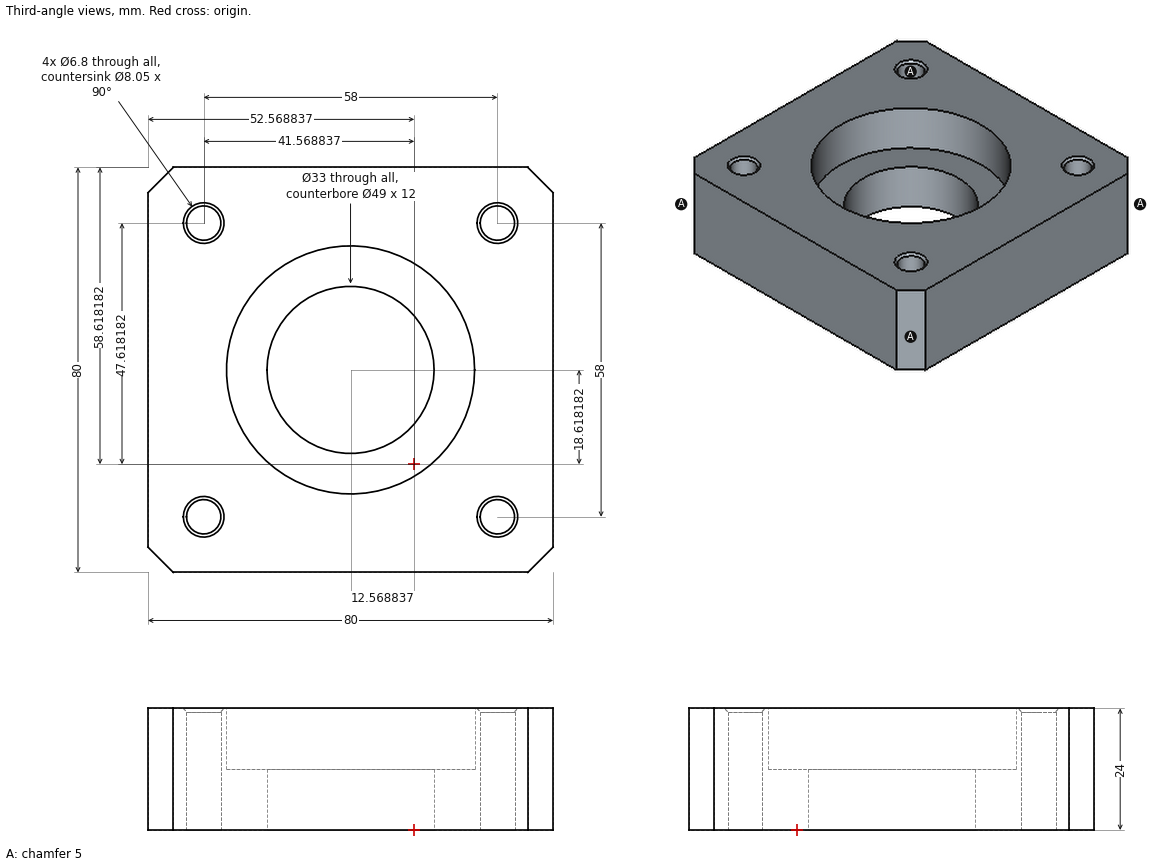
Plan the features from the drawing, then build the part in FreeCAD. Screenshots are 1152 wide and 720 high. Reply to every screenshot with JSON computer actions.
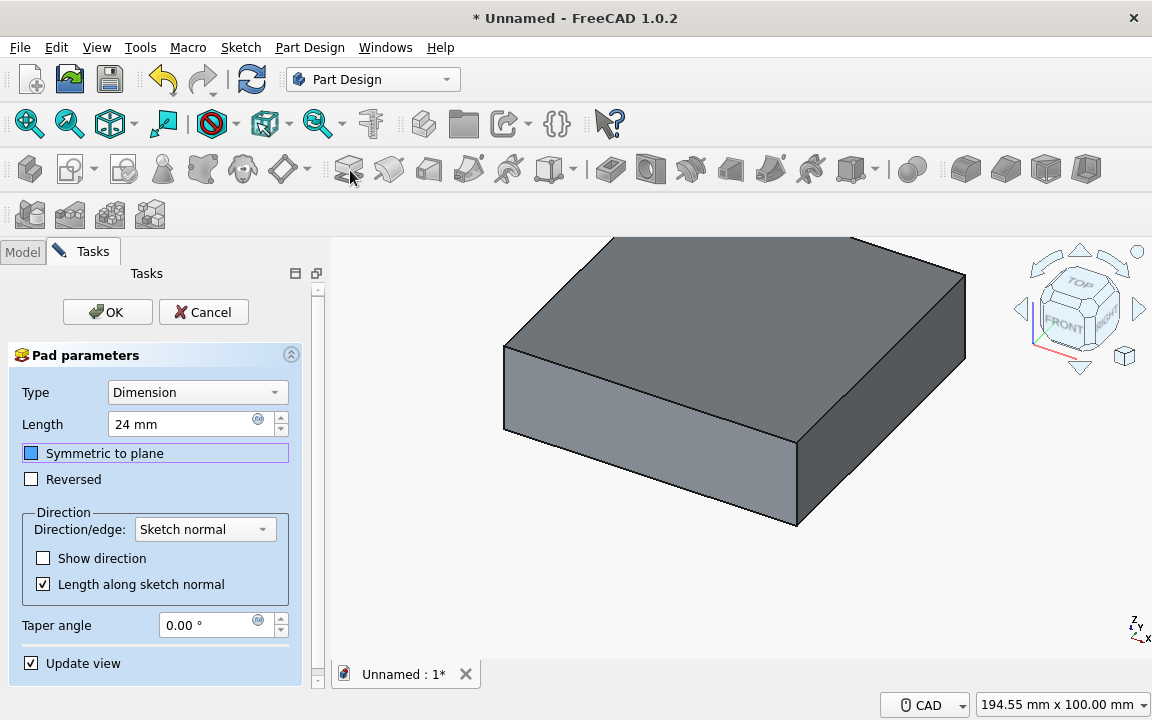
{"action": "left_click", "coordinate": [108, 312]}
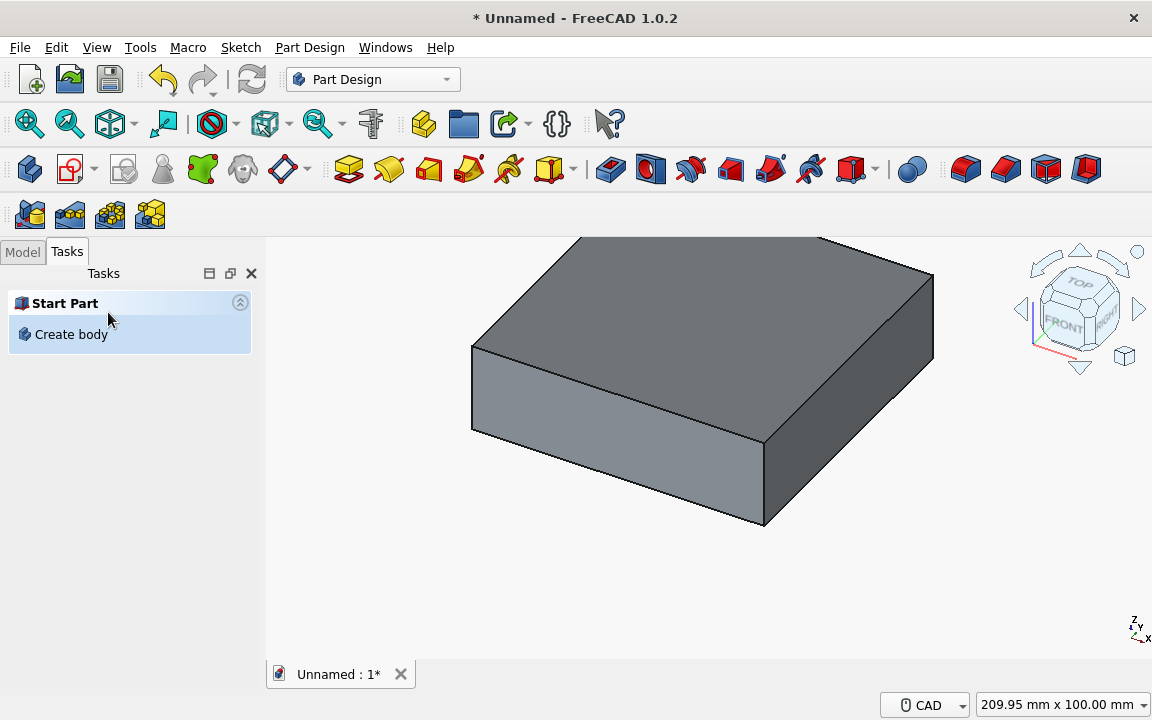
{"action": "key", "text": "v f"}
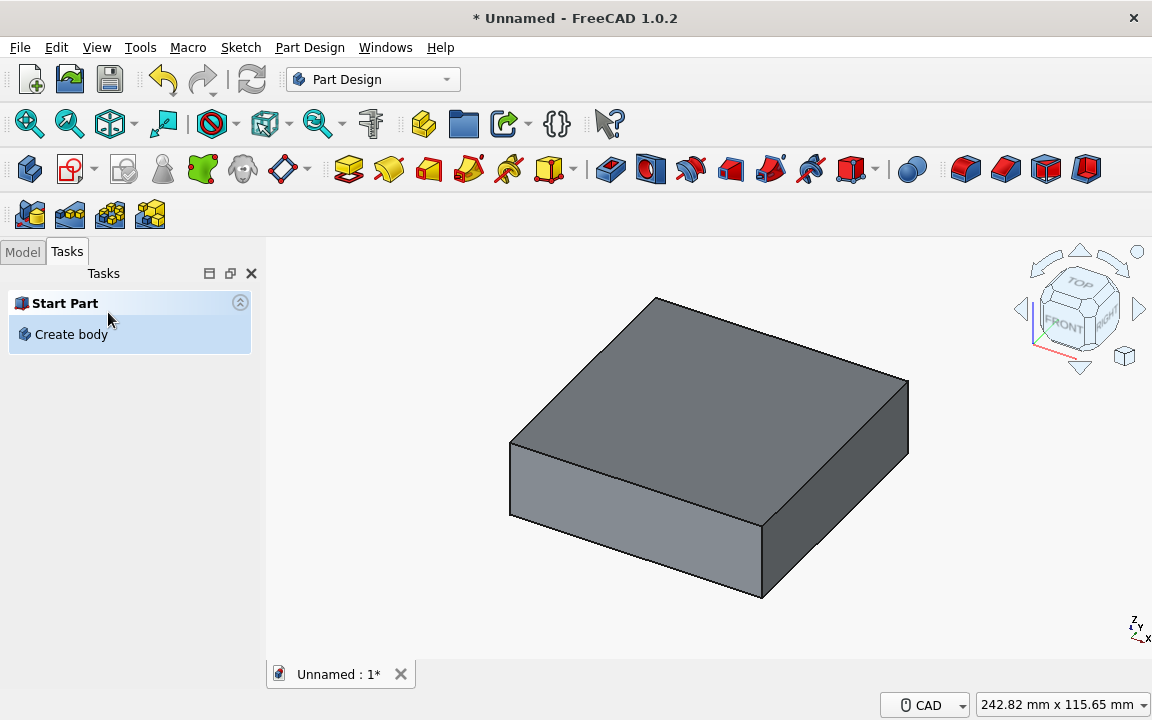
{"action": "left_click", "coordinate": [709, 411]}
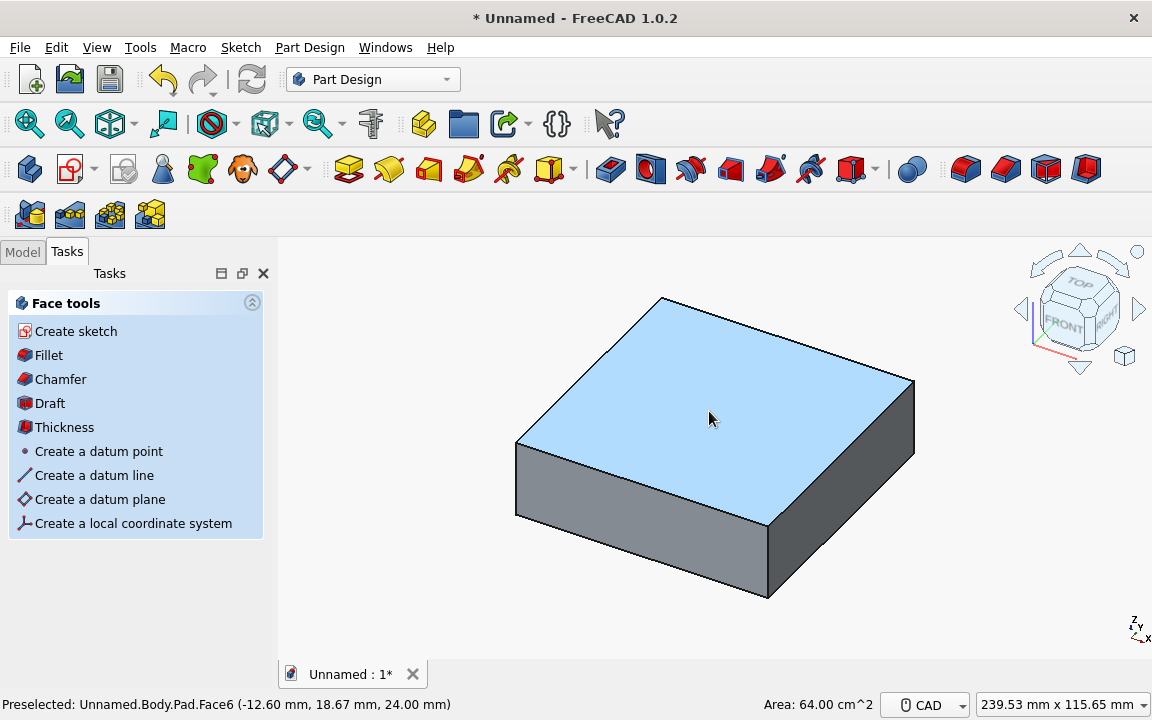
{"action": "left_click", "coordinate": [70, 170]}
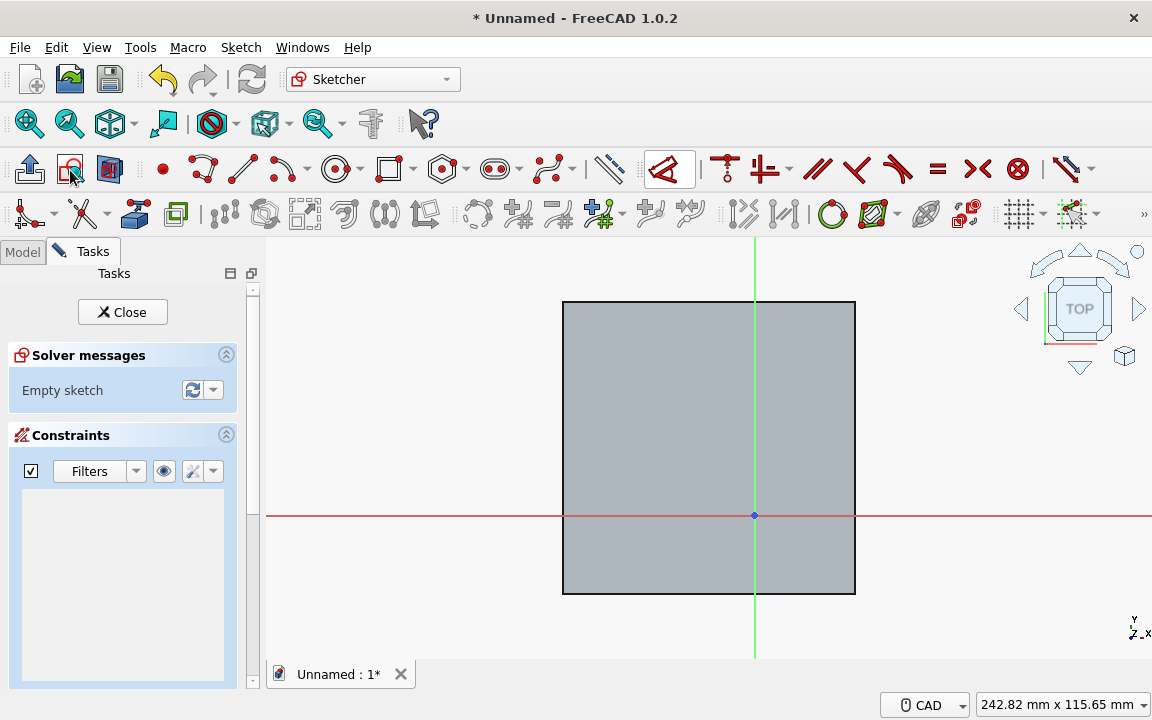
{"action": "scroll", "coordinate": [765, 455], "scroll_direction": "up", "scroll_amount": 4}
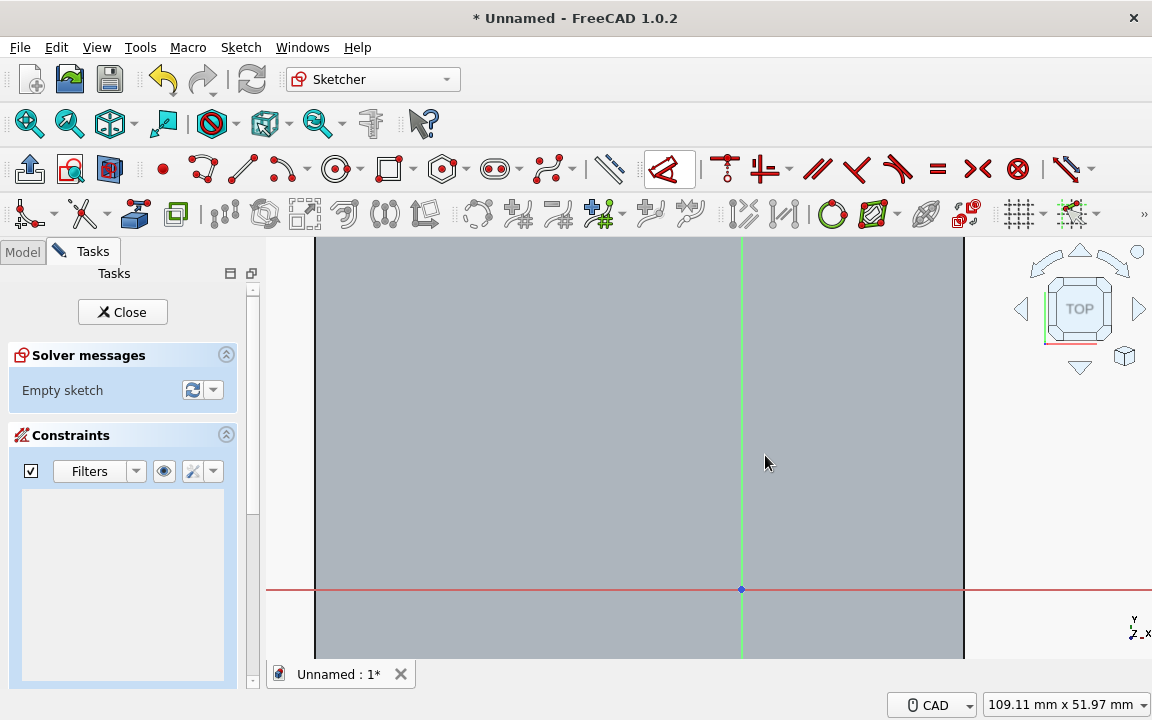
{"action": "key", "text": "g c"}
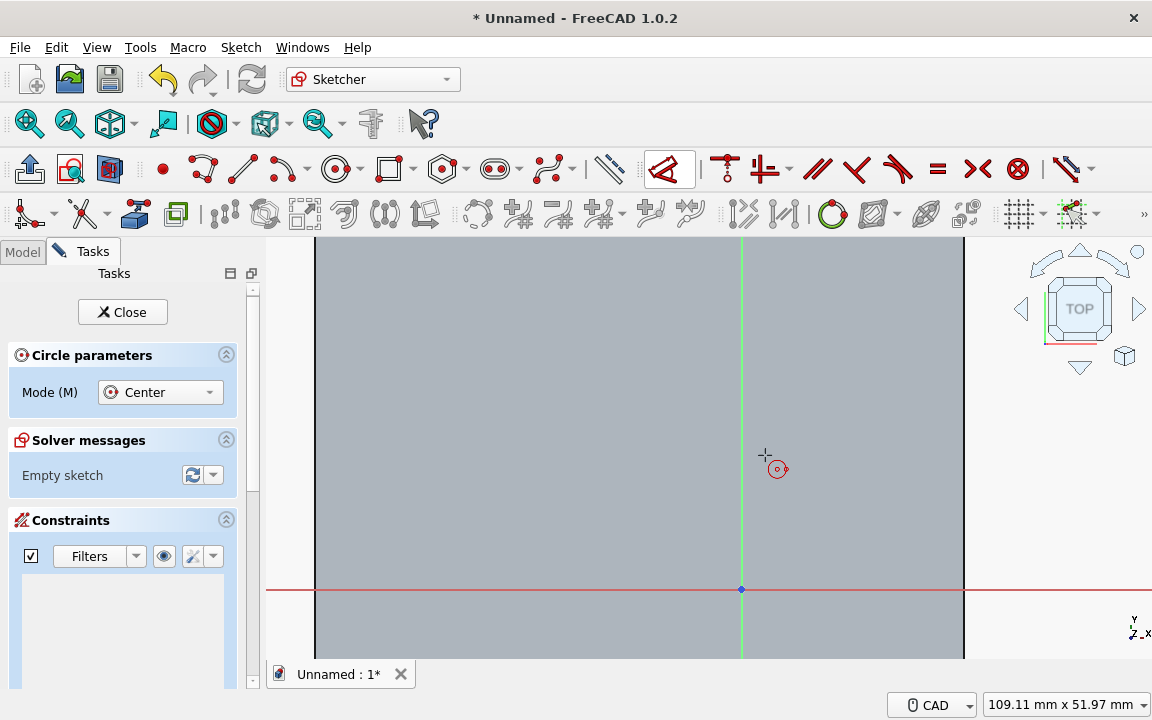
{"action": "left_click", "coordinate": [640, 439]}
{"action": "left_click", "coordinate": [545, 344]}
{"action": "key", "text": "Escape"}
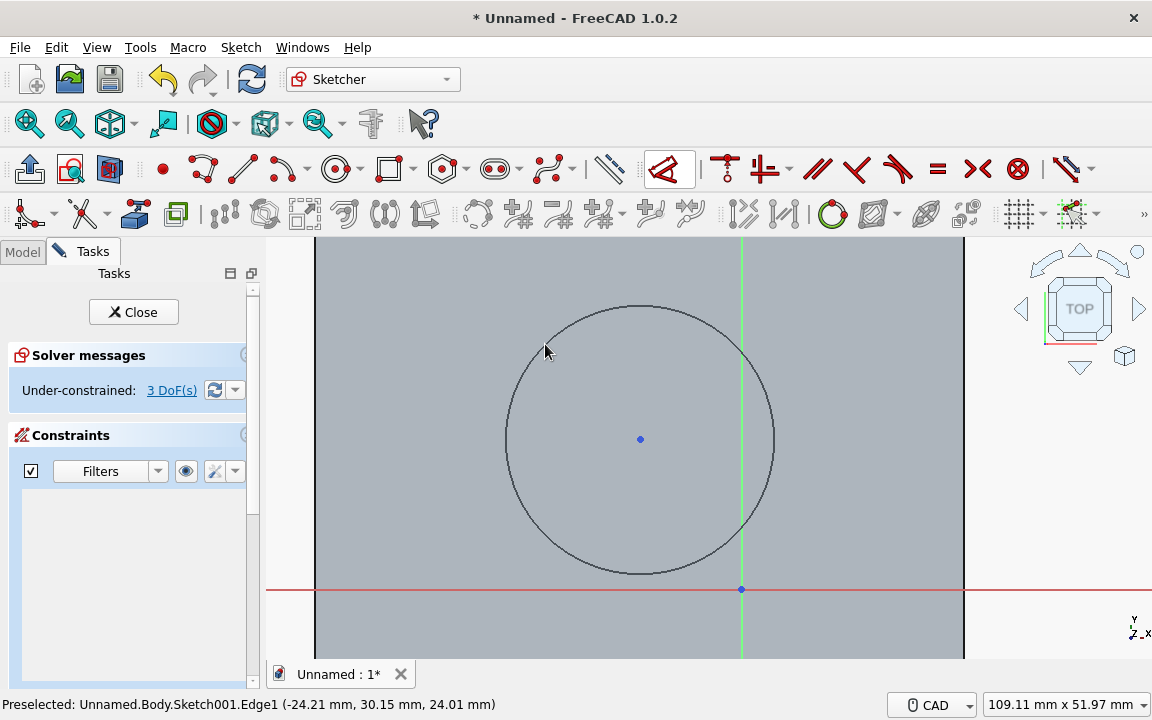
{"action": "left_click", "coordinate": [545, 345]}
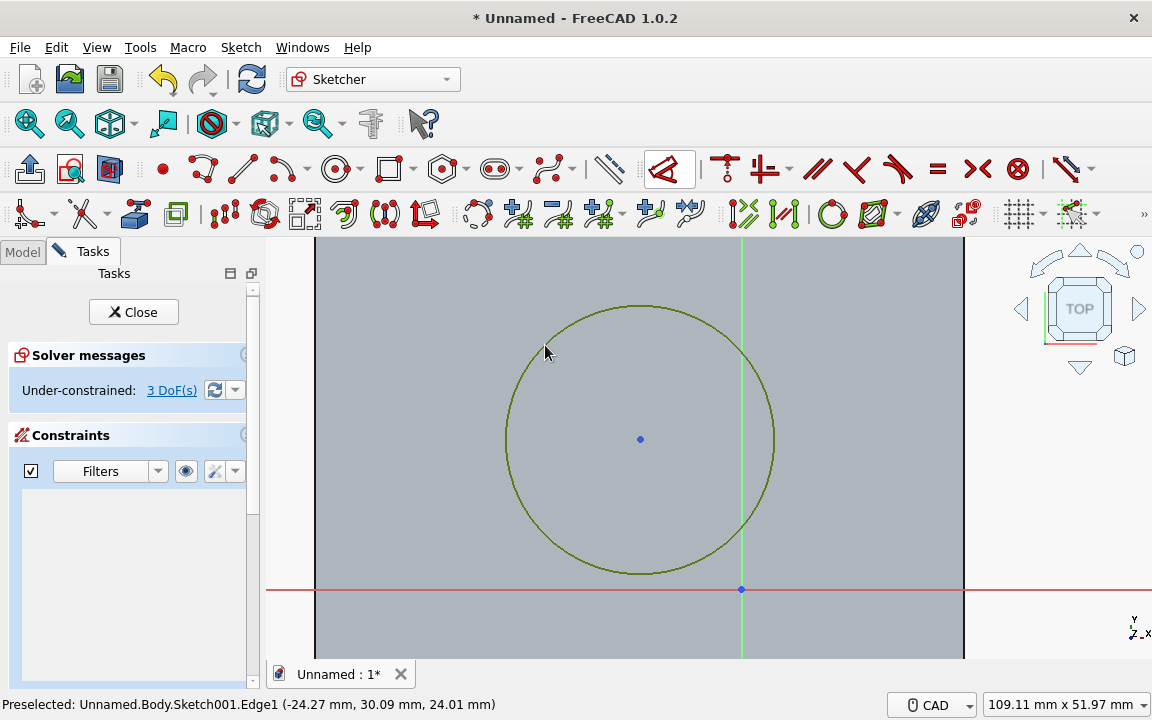
{"action": "key", "text": "k o"}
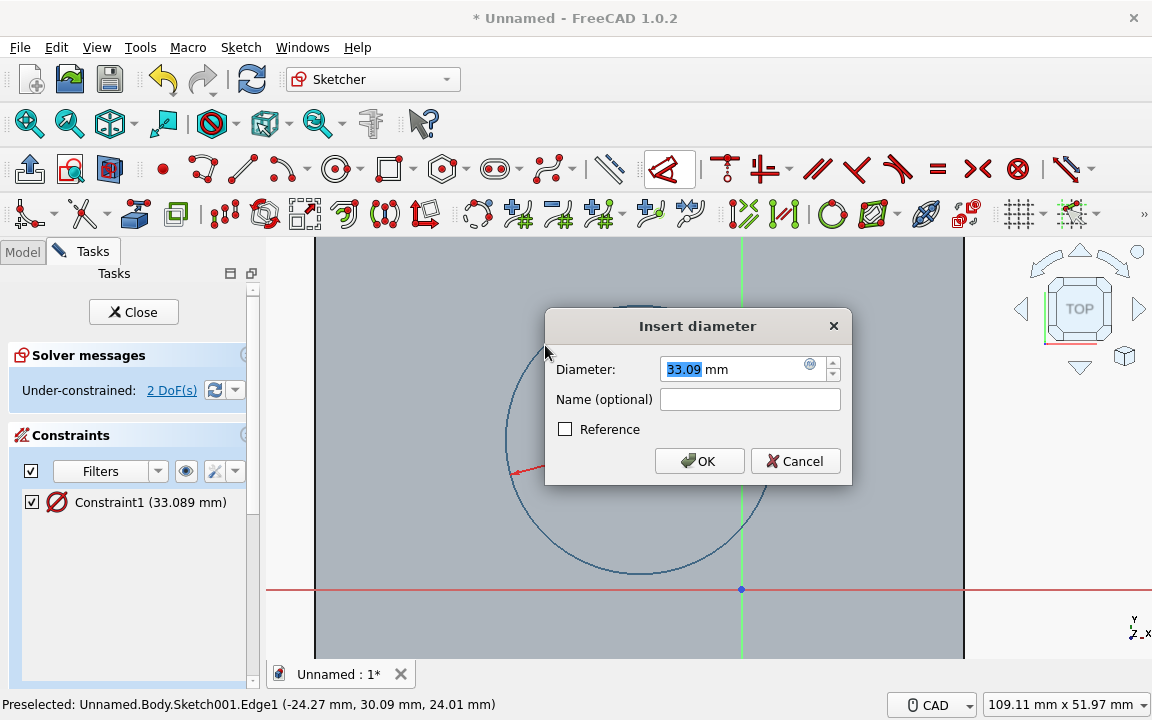
{"action": "type", "text": "33"}
{"action": "key", "text": "Return"}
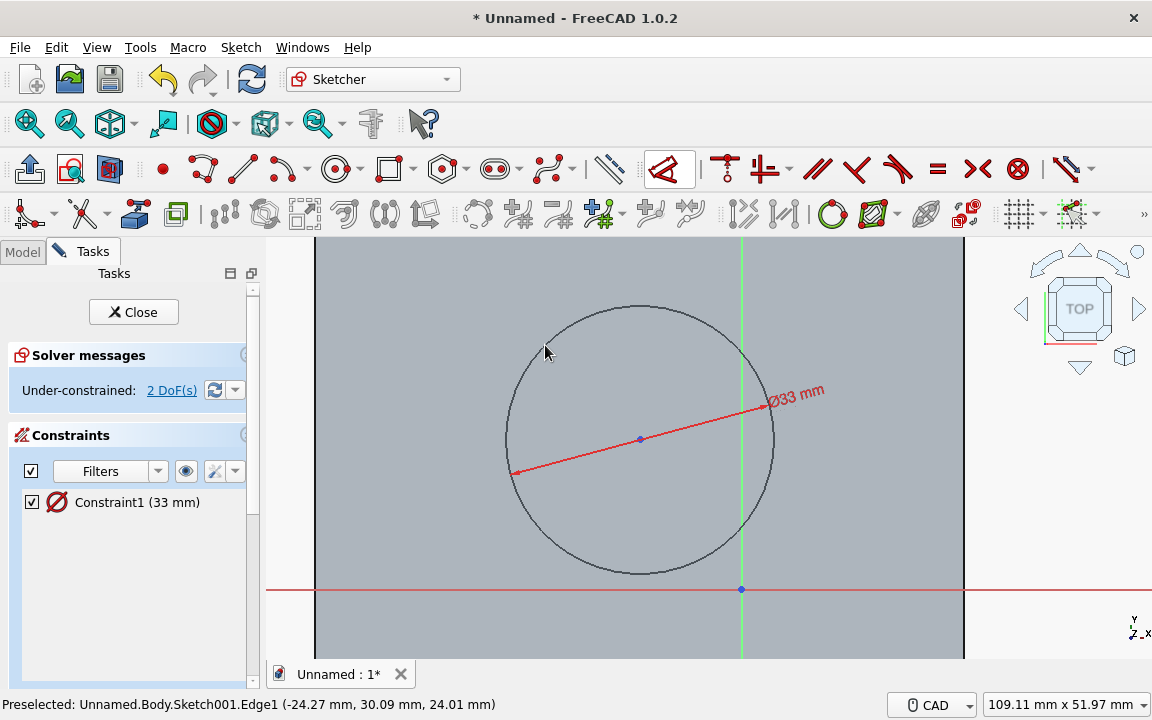
{"action": "left_click", "coordinate": [640, 440]}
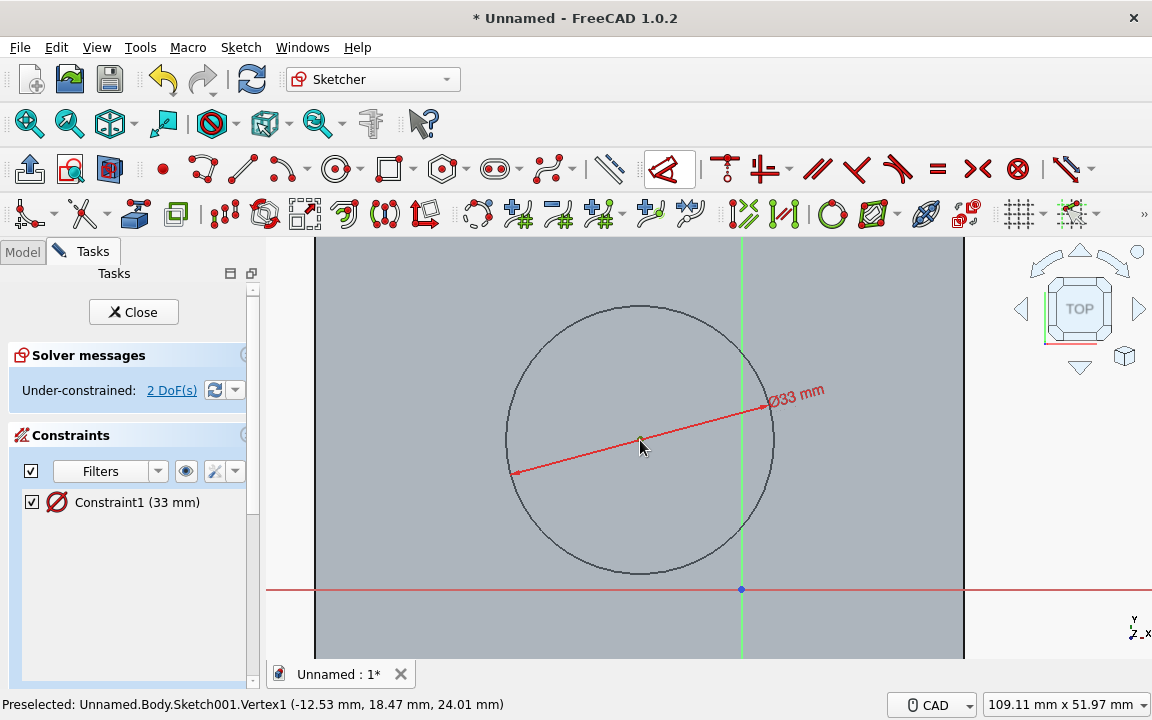
{"action": "key", "text": "l"}